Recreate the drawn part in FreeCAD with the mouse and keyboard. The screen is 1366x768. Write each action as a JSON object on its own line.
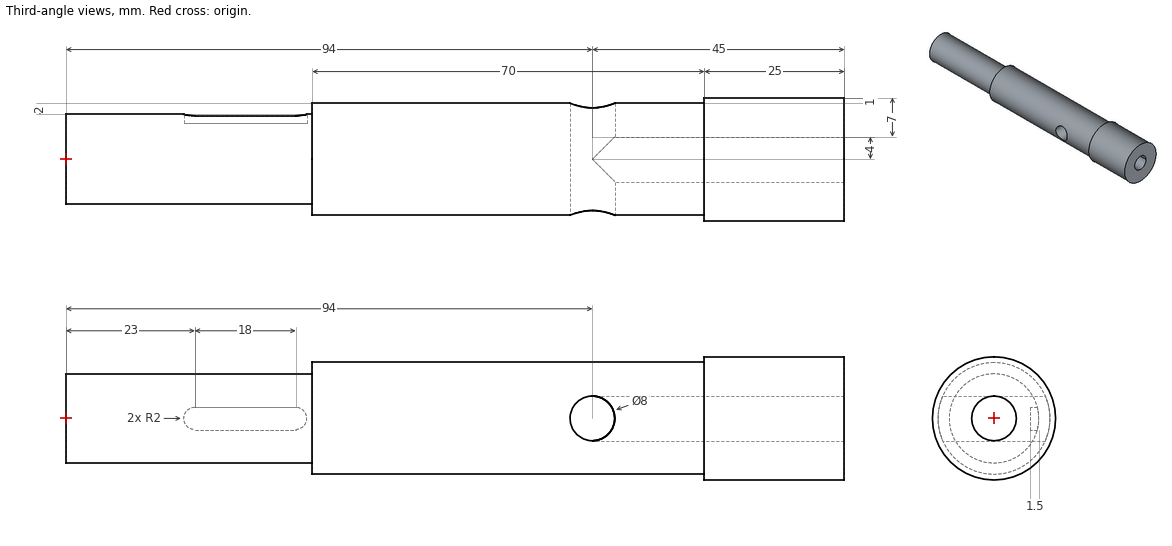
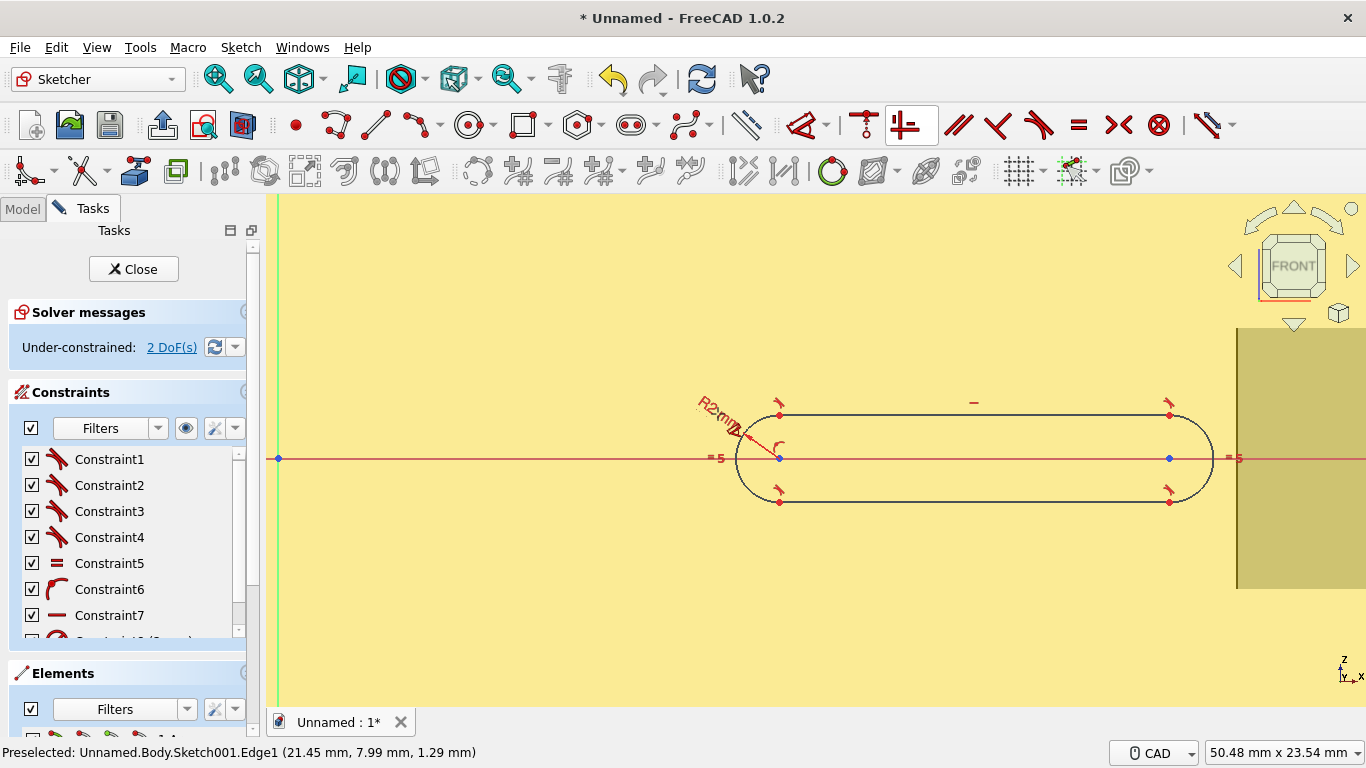
{"action": "left_click", "coordinate": [897, 415]}
{"action": "left_click", "coordinate": [975, 381]}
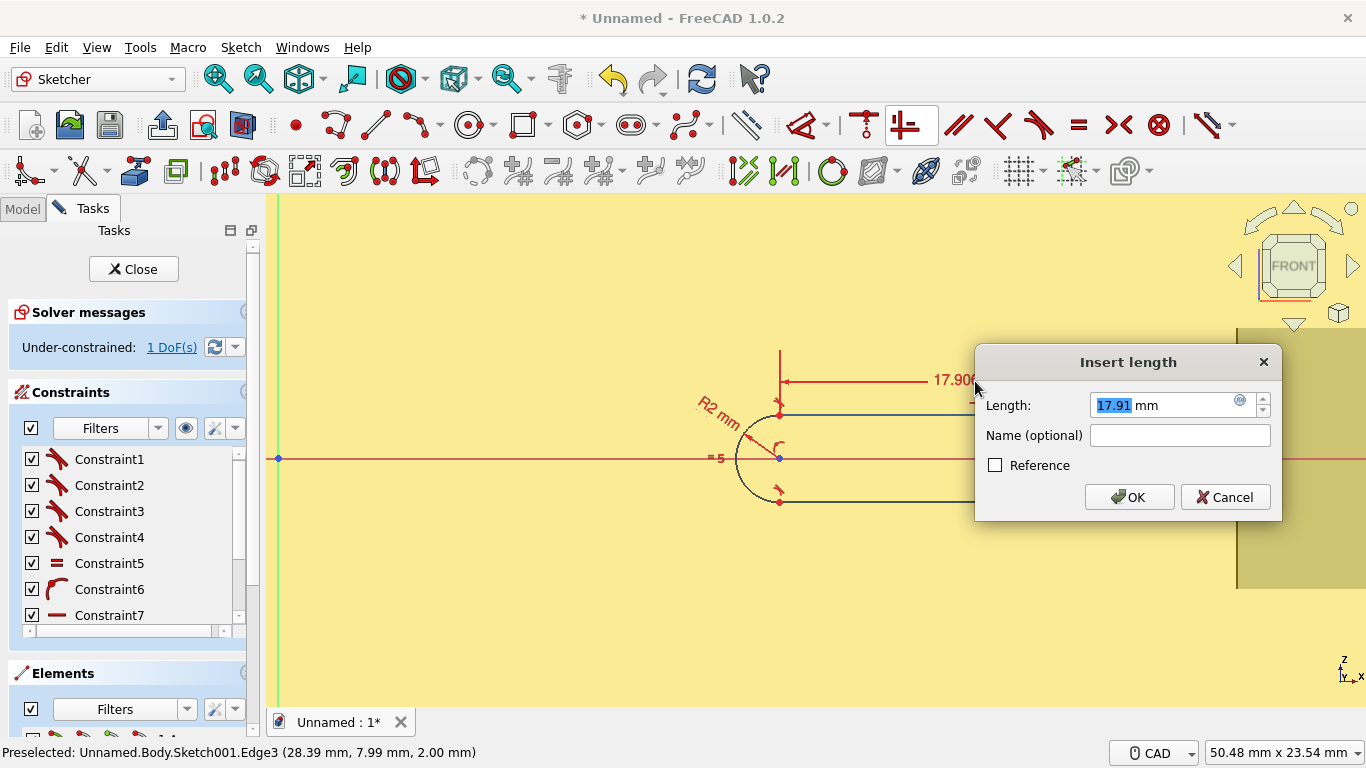
{"action": "type", "text": "18"}
{"action": "key", "text": "Return"}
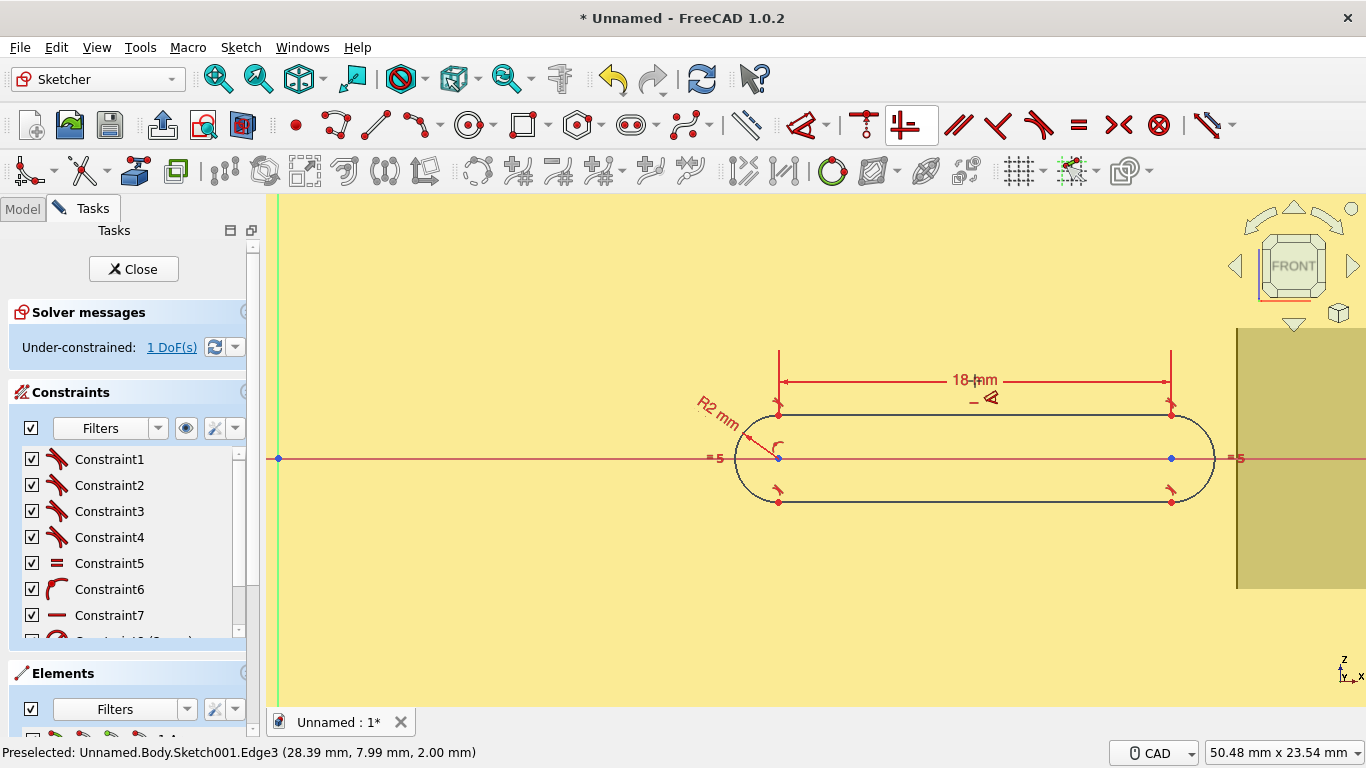
{"action": "left_click", "coordinate": [779, 415]}
{"action": "left_click", "coordinate": [536, 381]}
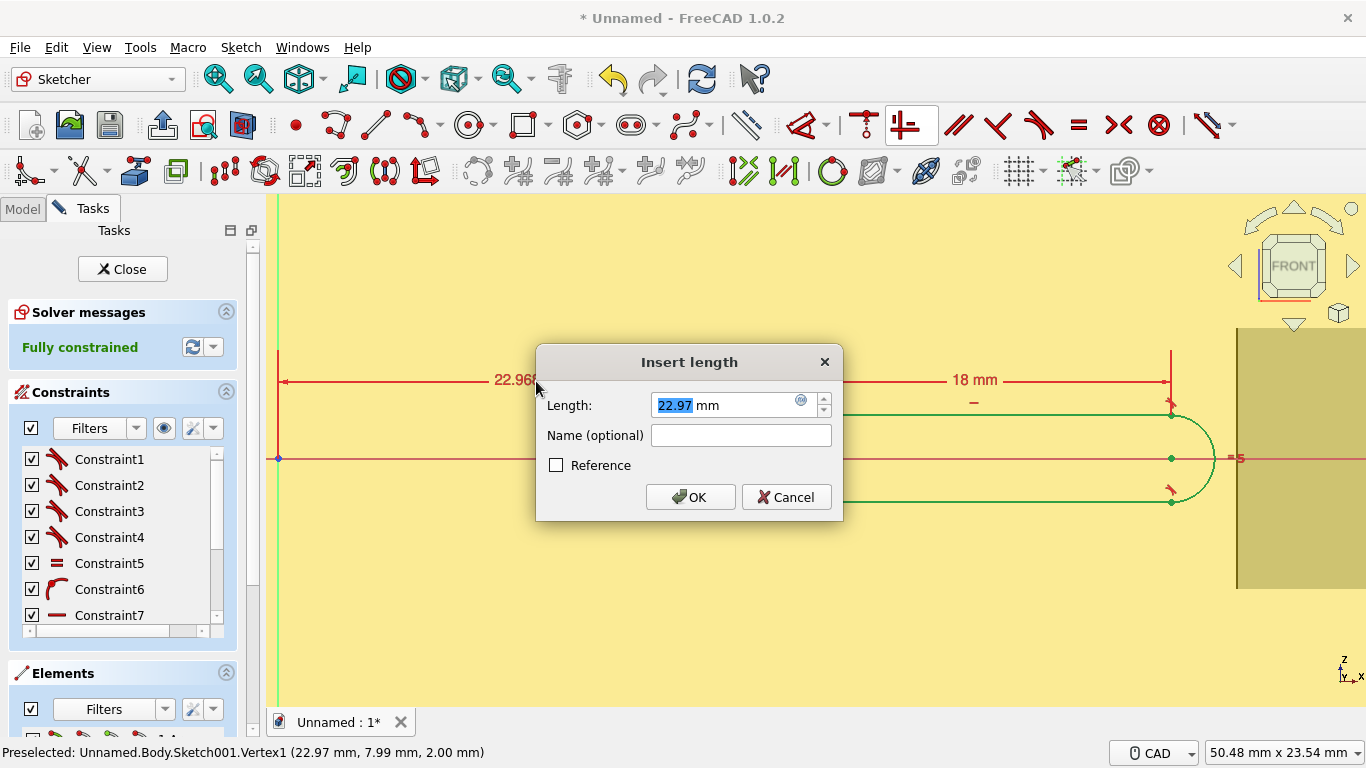
{"action": "type", "text": "23"}
{"action": "key", "text": "Return"}
{"action": "key", "text": "Escape"}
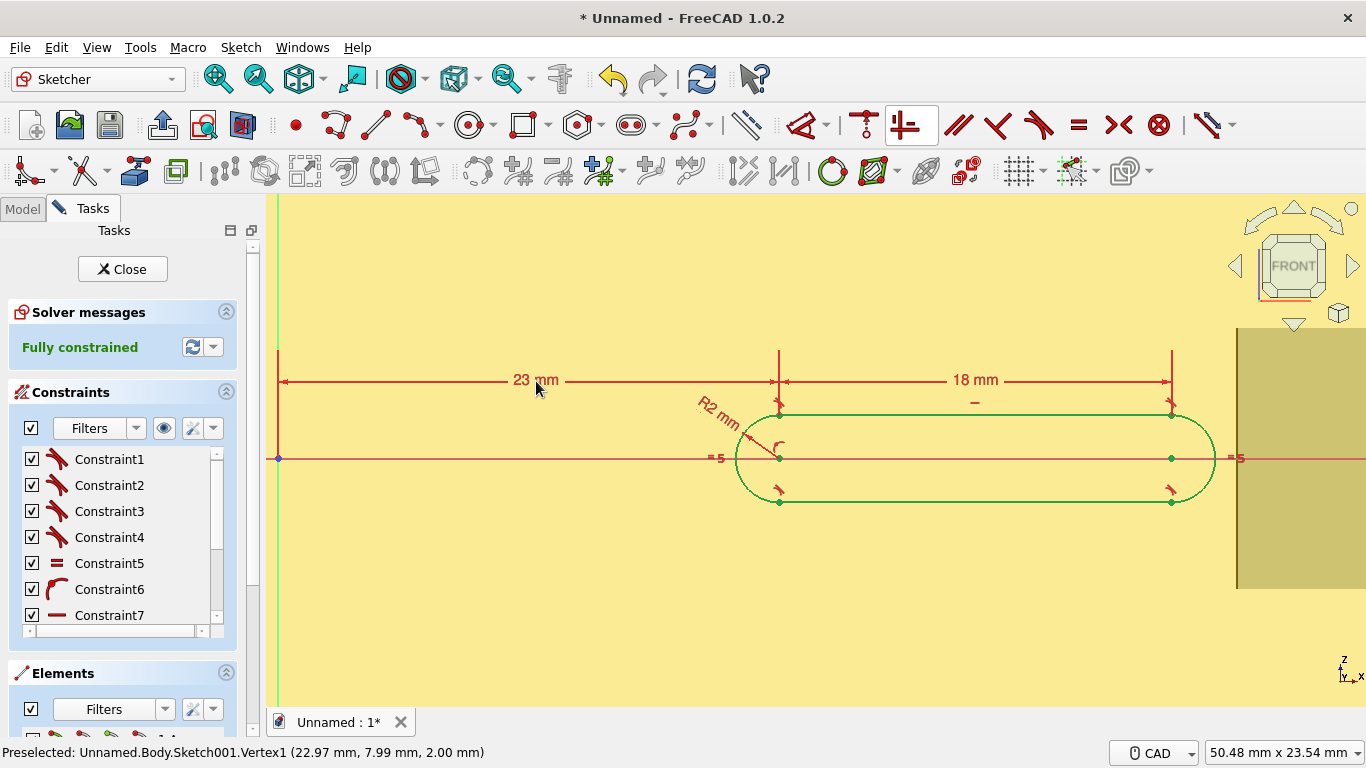
{"action": "left_click", "coordinate": [123, 269]}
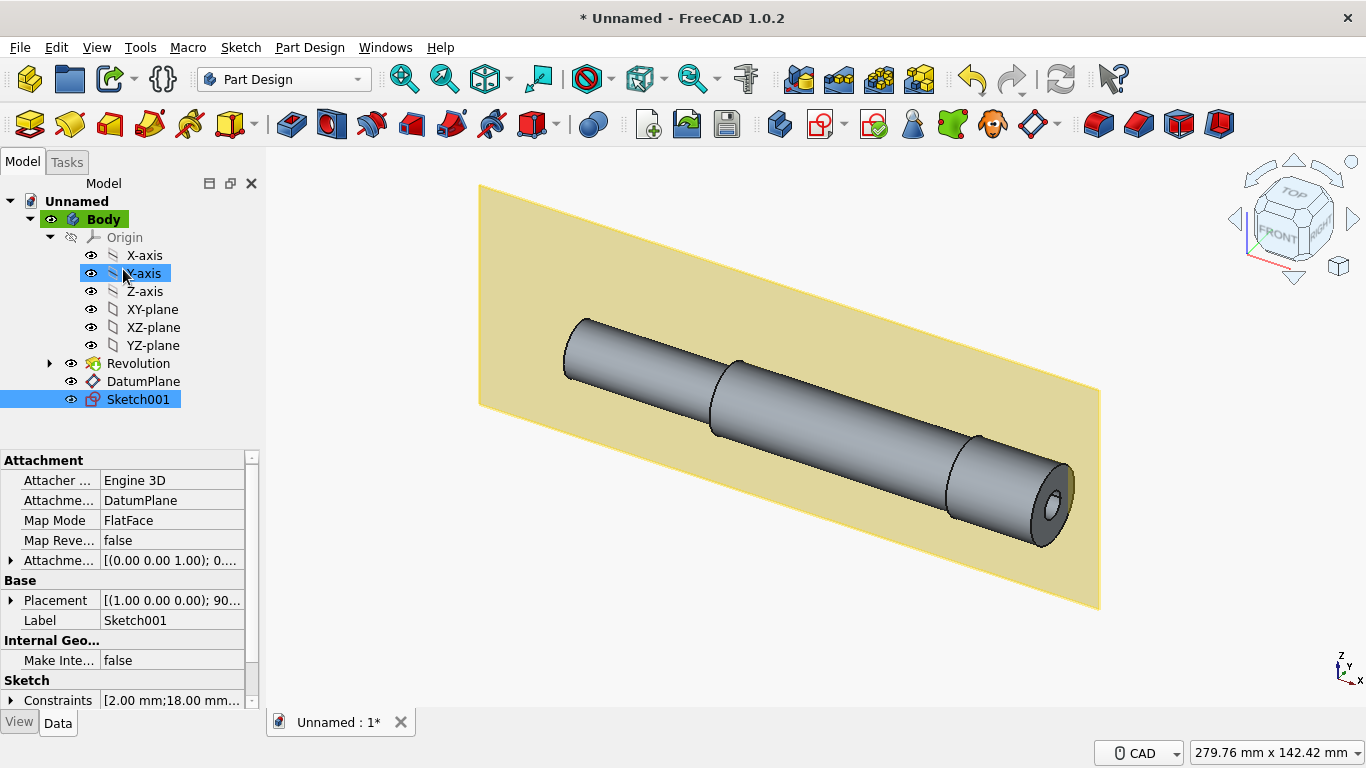
{"action": "left_click", "coordinate": [292, 124]}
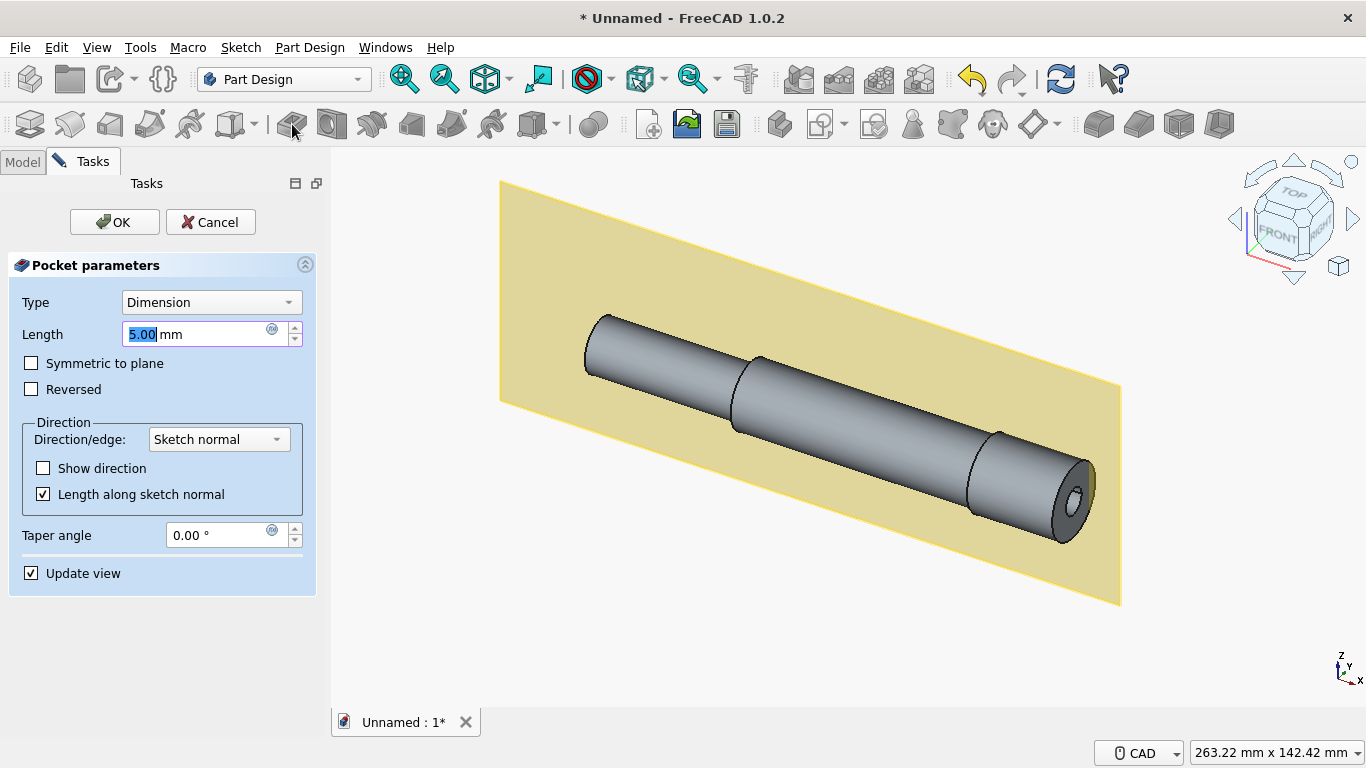
{"action": "type", "text": "1.5"}
{"action": "key", "text": "Tab"}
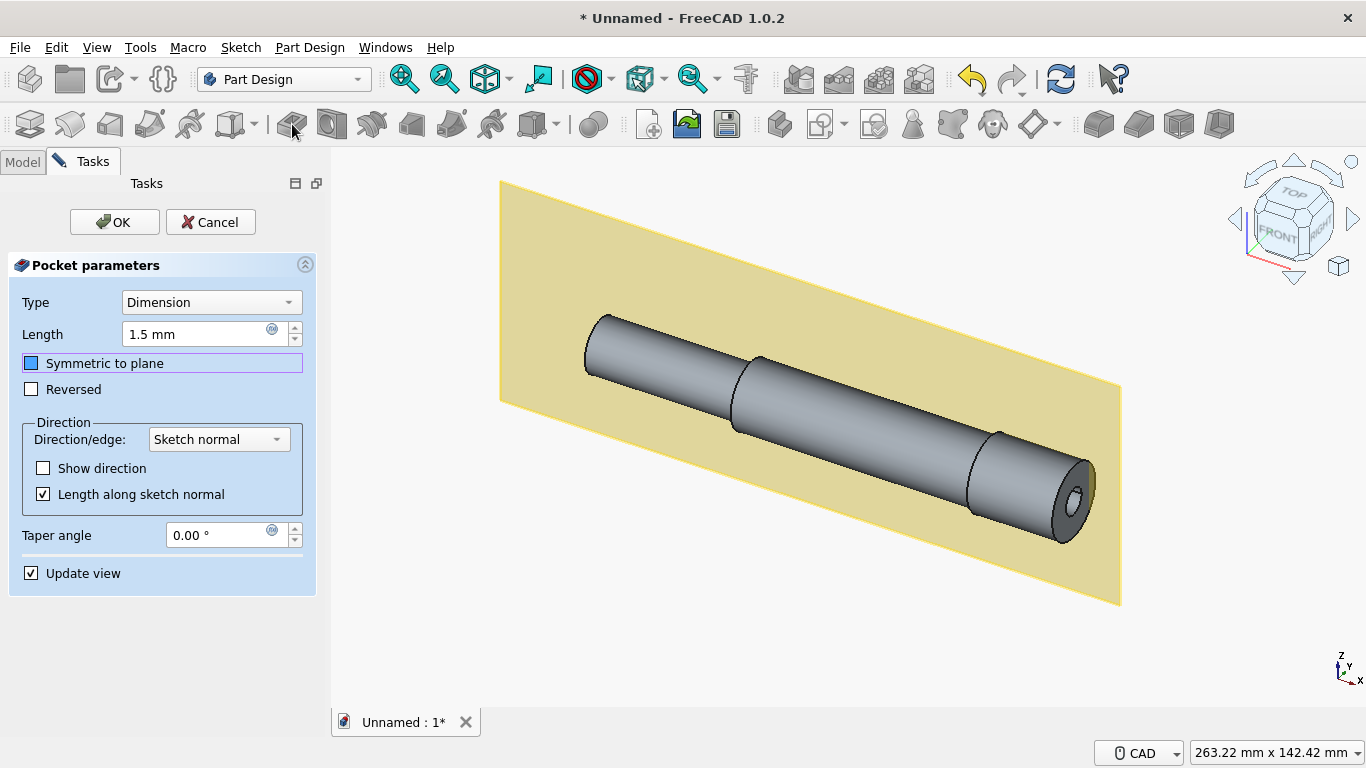
{"action": "left_click", "coordinate": [30, 389]}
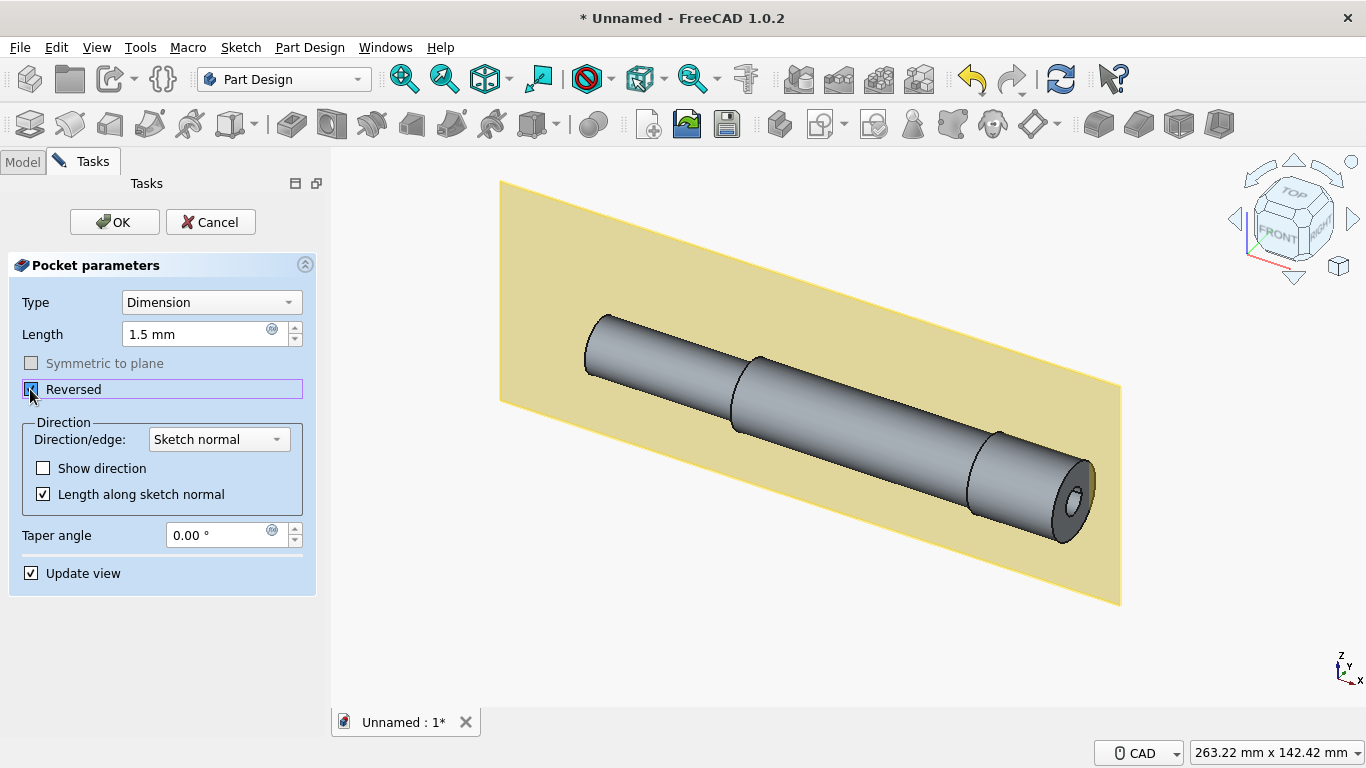
{"action": "left_click", "coordinate": [115, 222]}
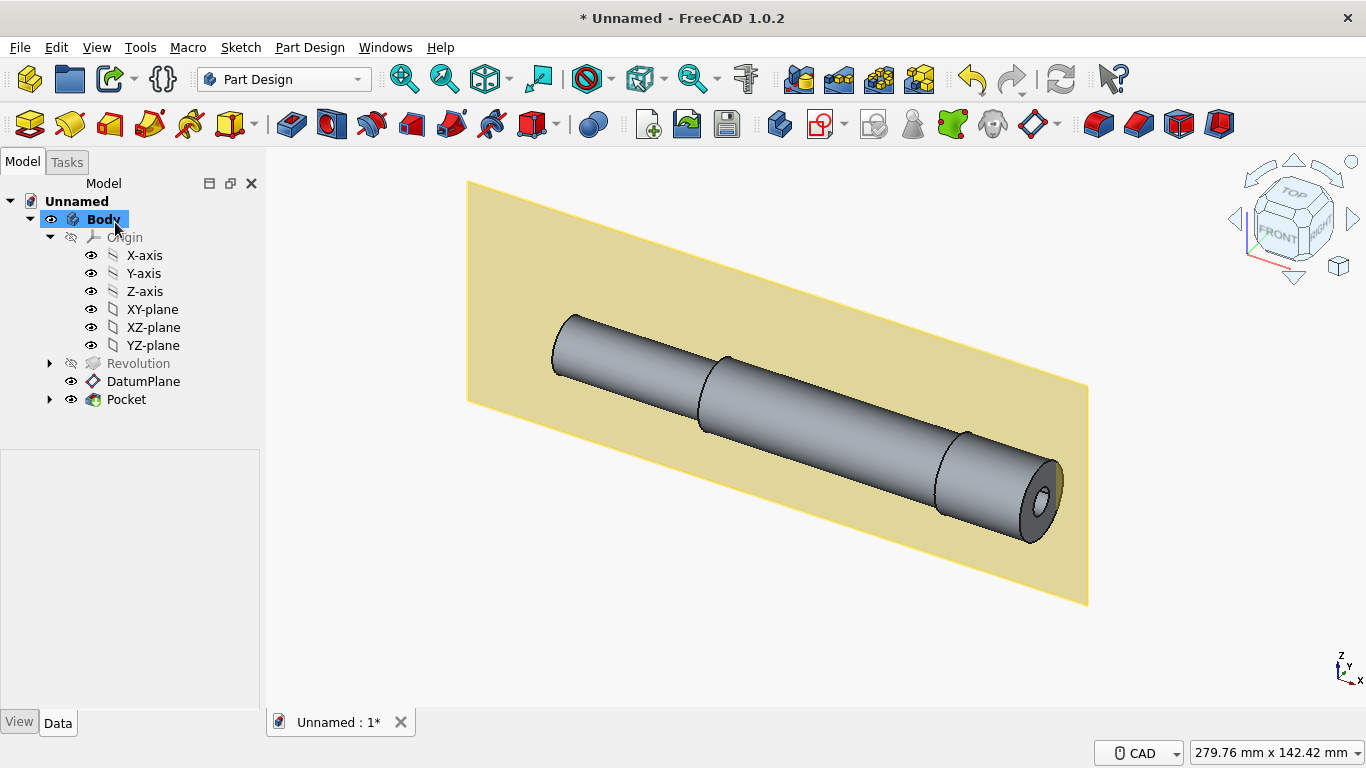
{"action": "left_click", "coordinate": [116, 381]}
{"action": "key", "text": "space"}